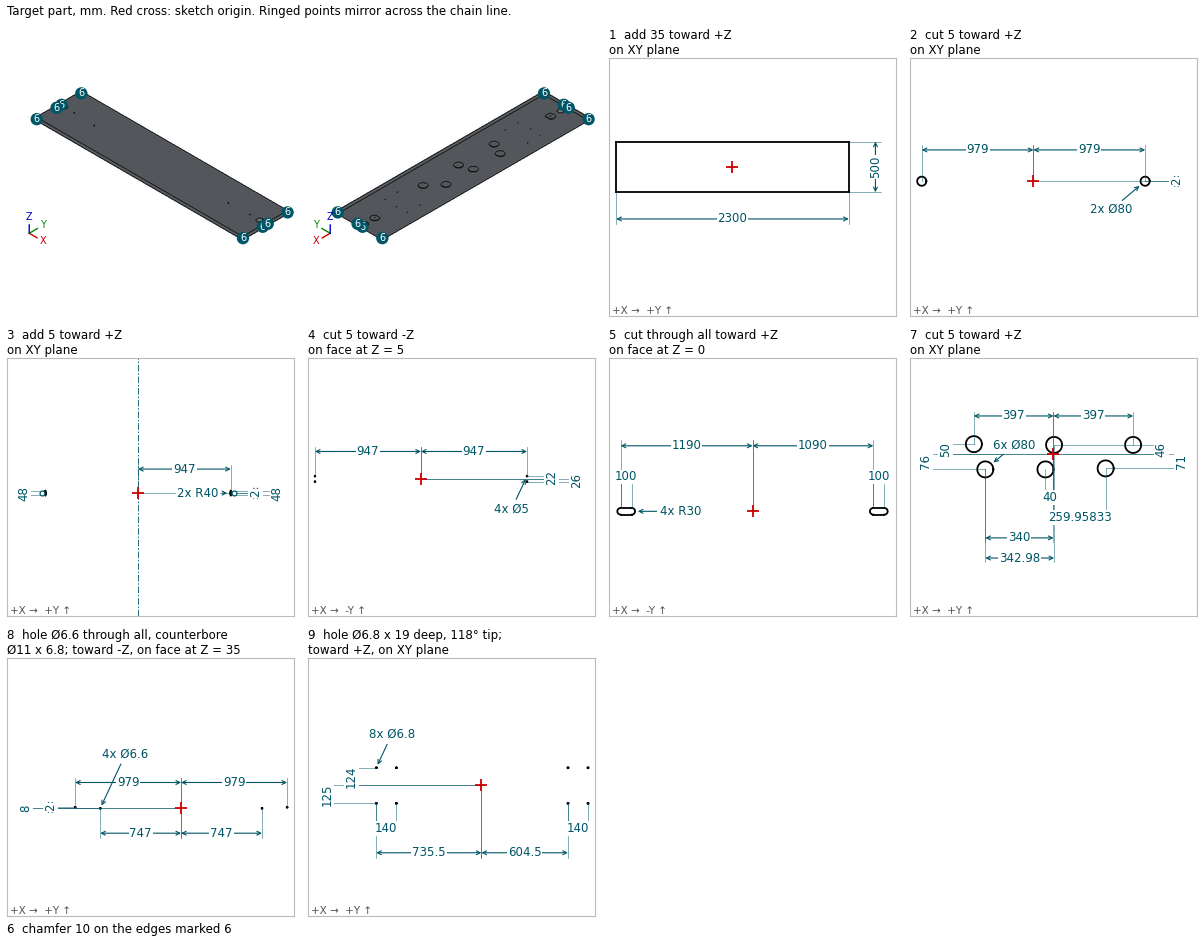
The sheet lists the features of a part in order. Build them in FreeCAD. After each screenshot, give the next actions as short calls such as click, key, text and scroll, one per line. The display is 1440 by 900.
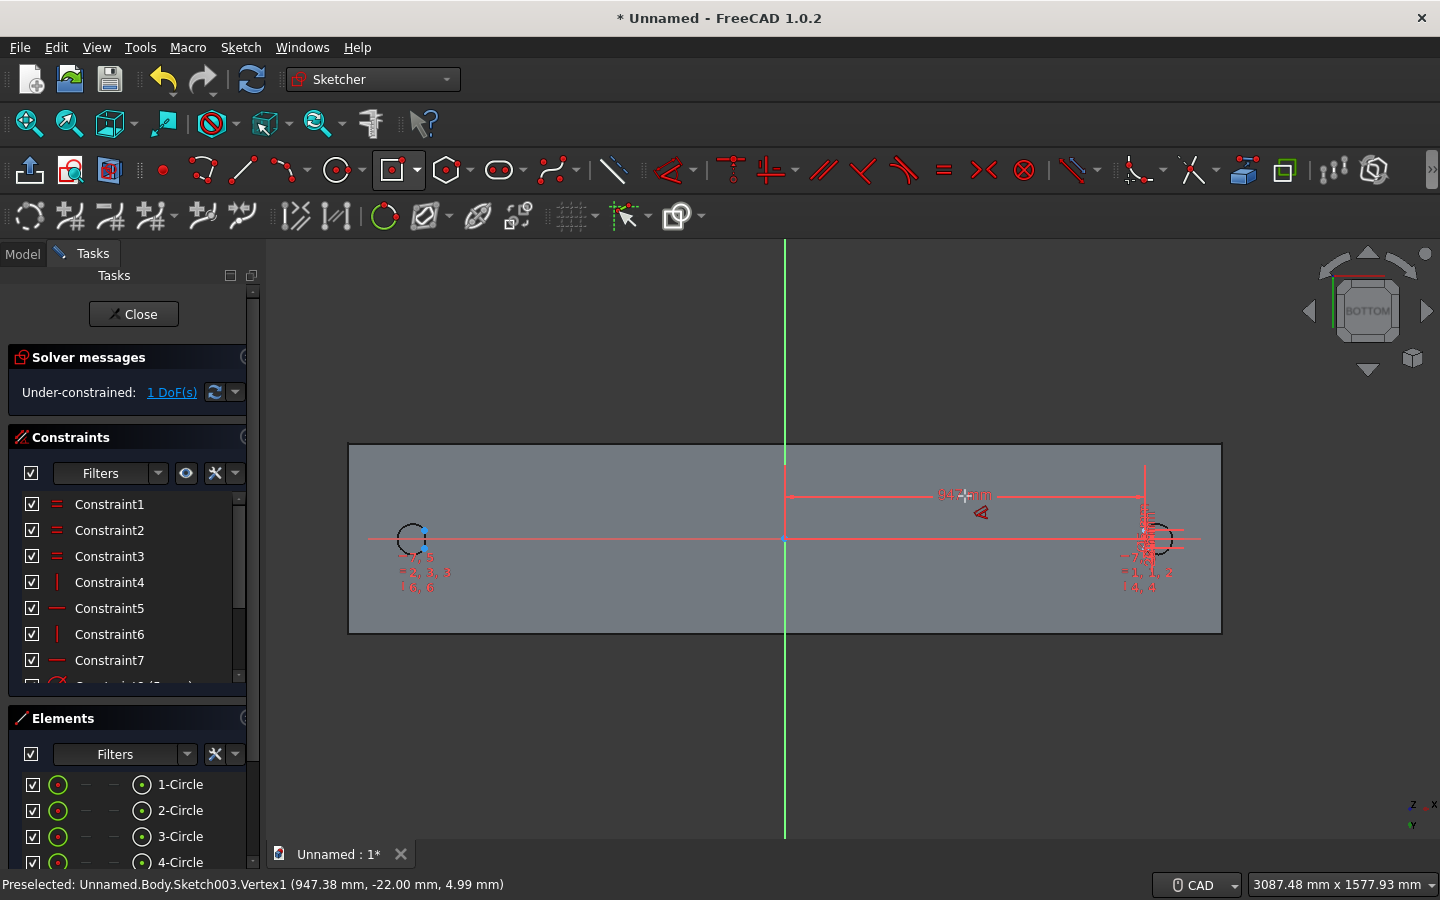
click(425, 530)
click(605, 496)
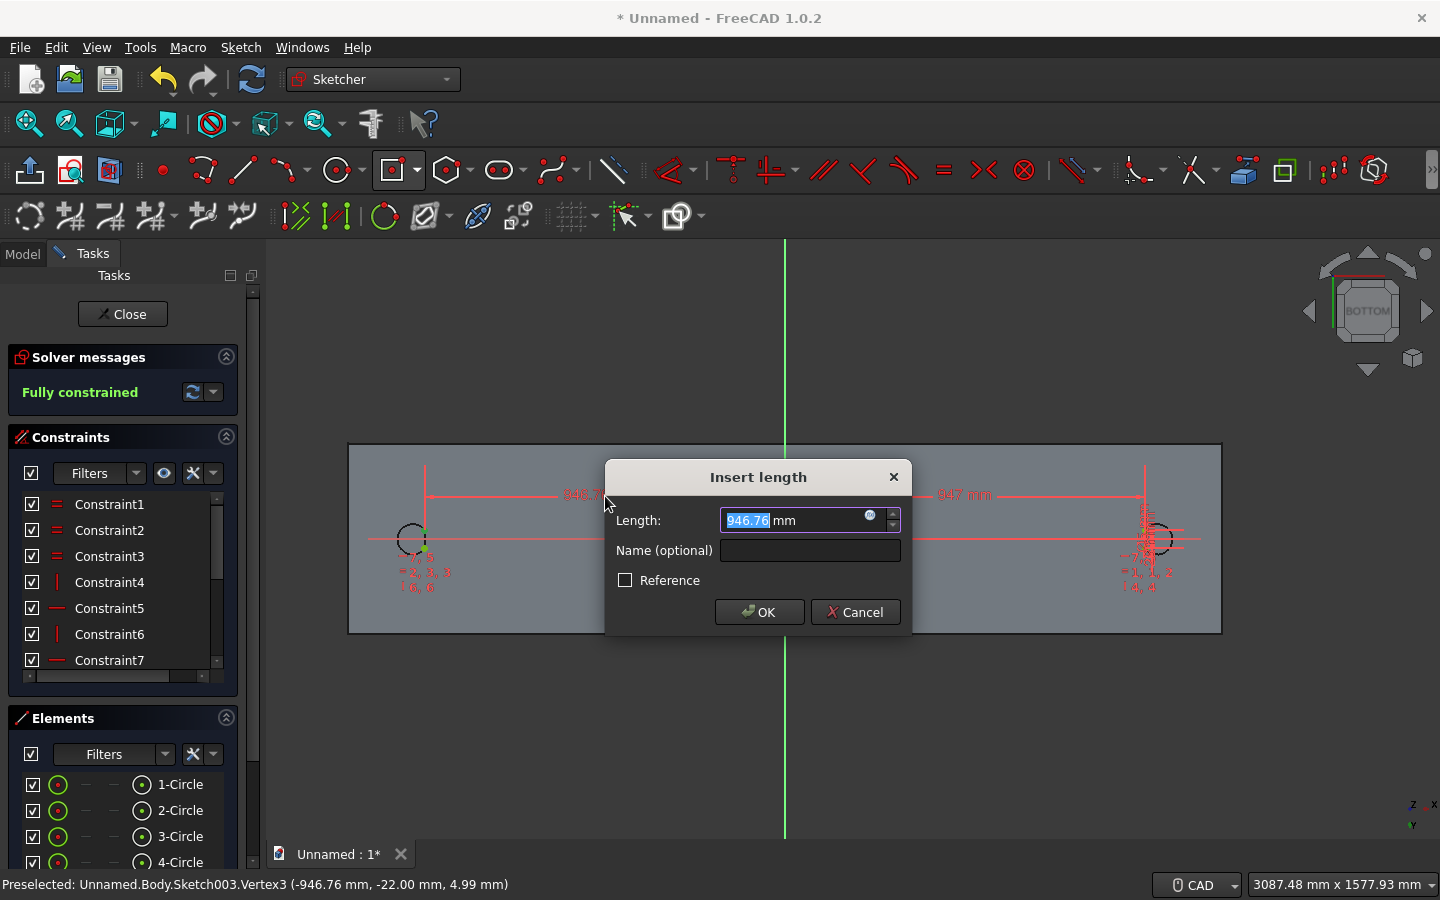
text(947)
key(Return)
key(Escape)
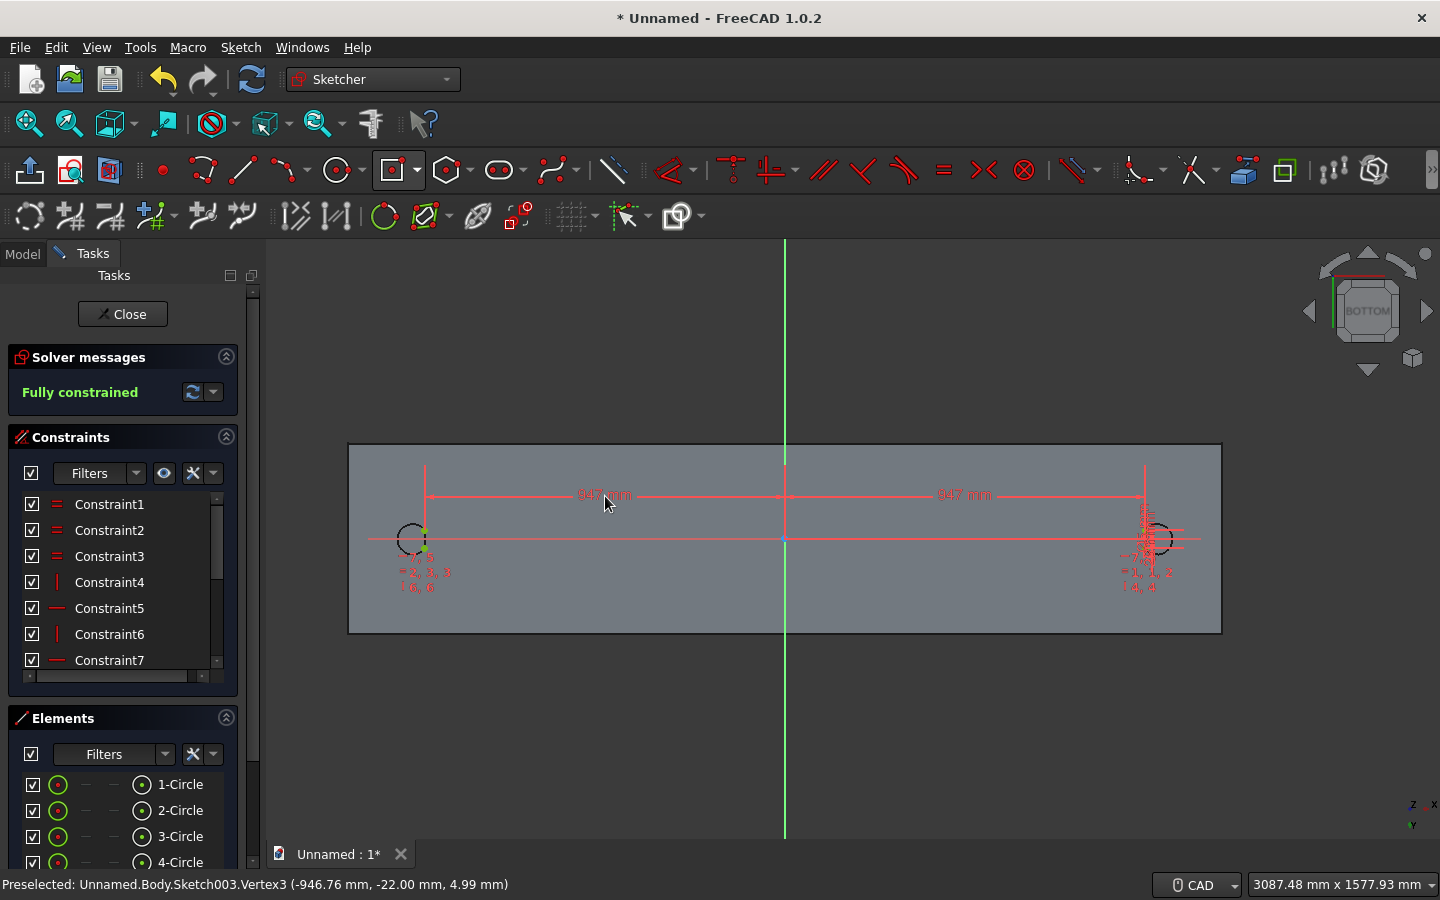
click(123, 314)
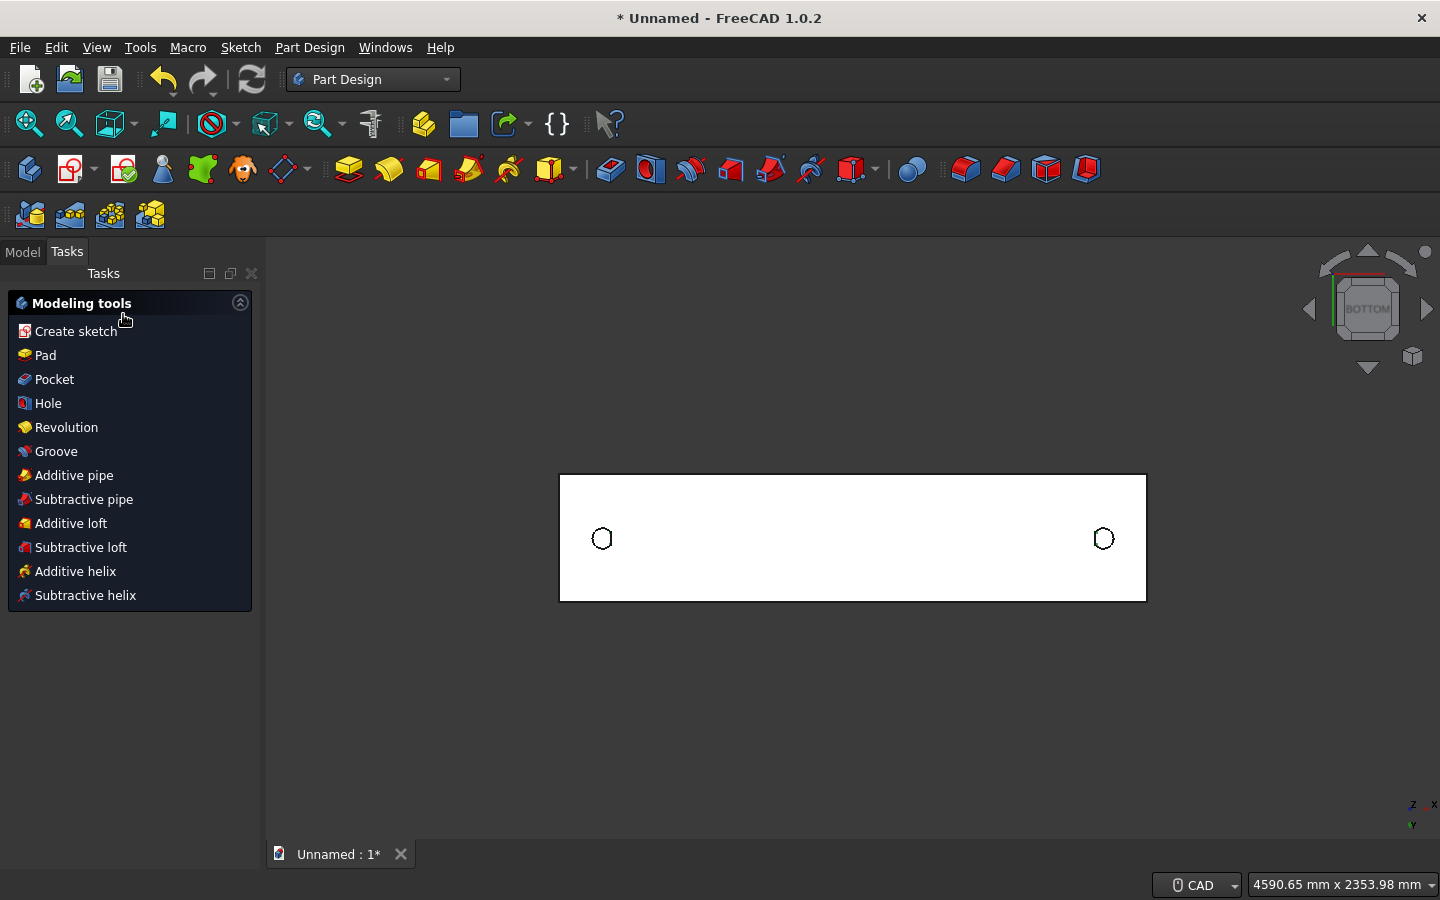
click(612, 170)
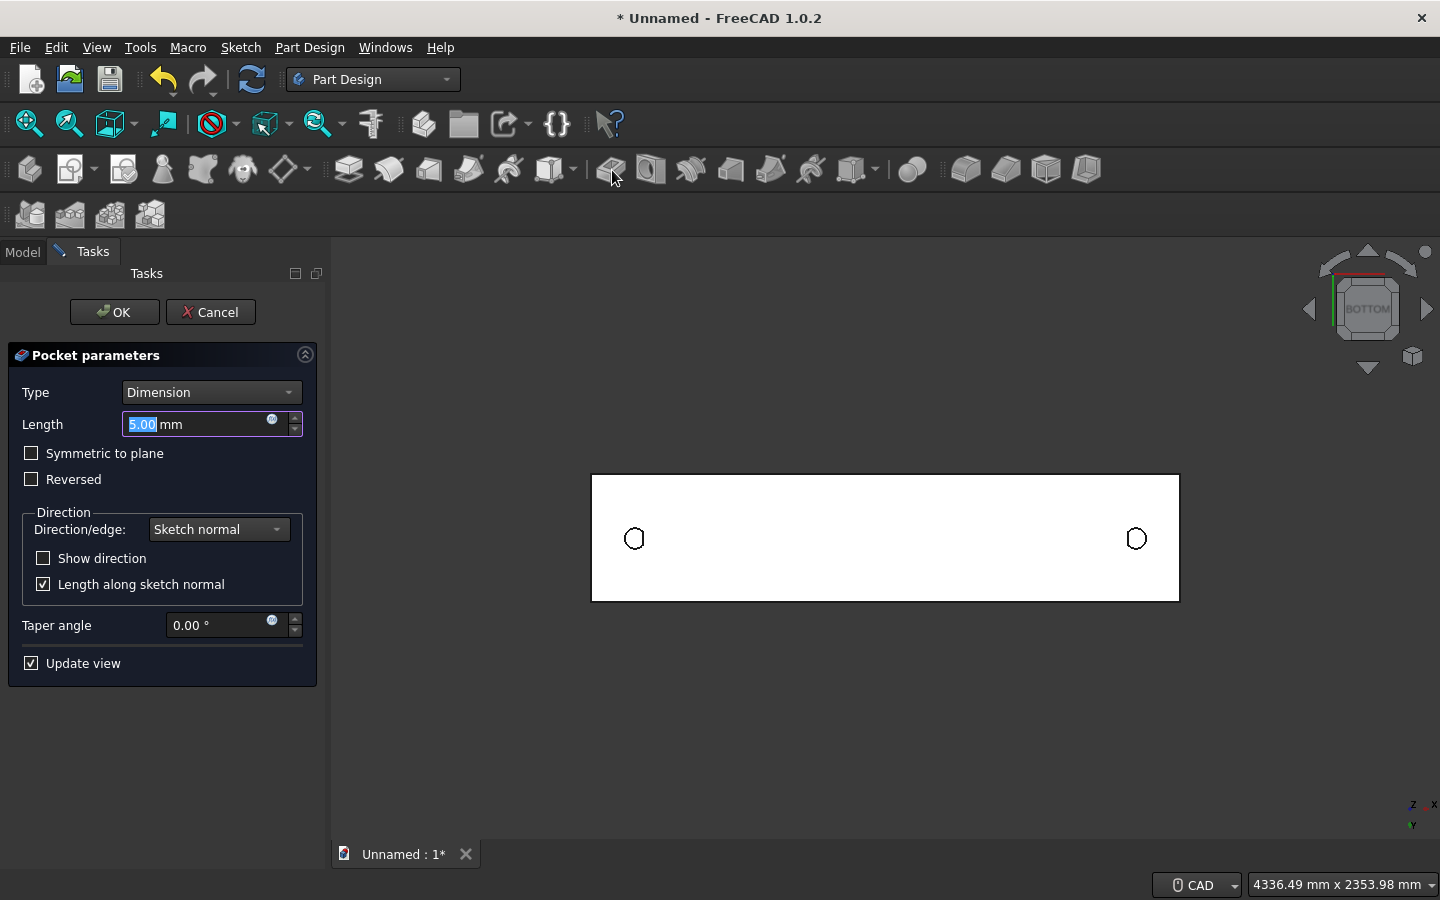
text(5)
key(Tab)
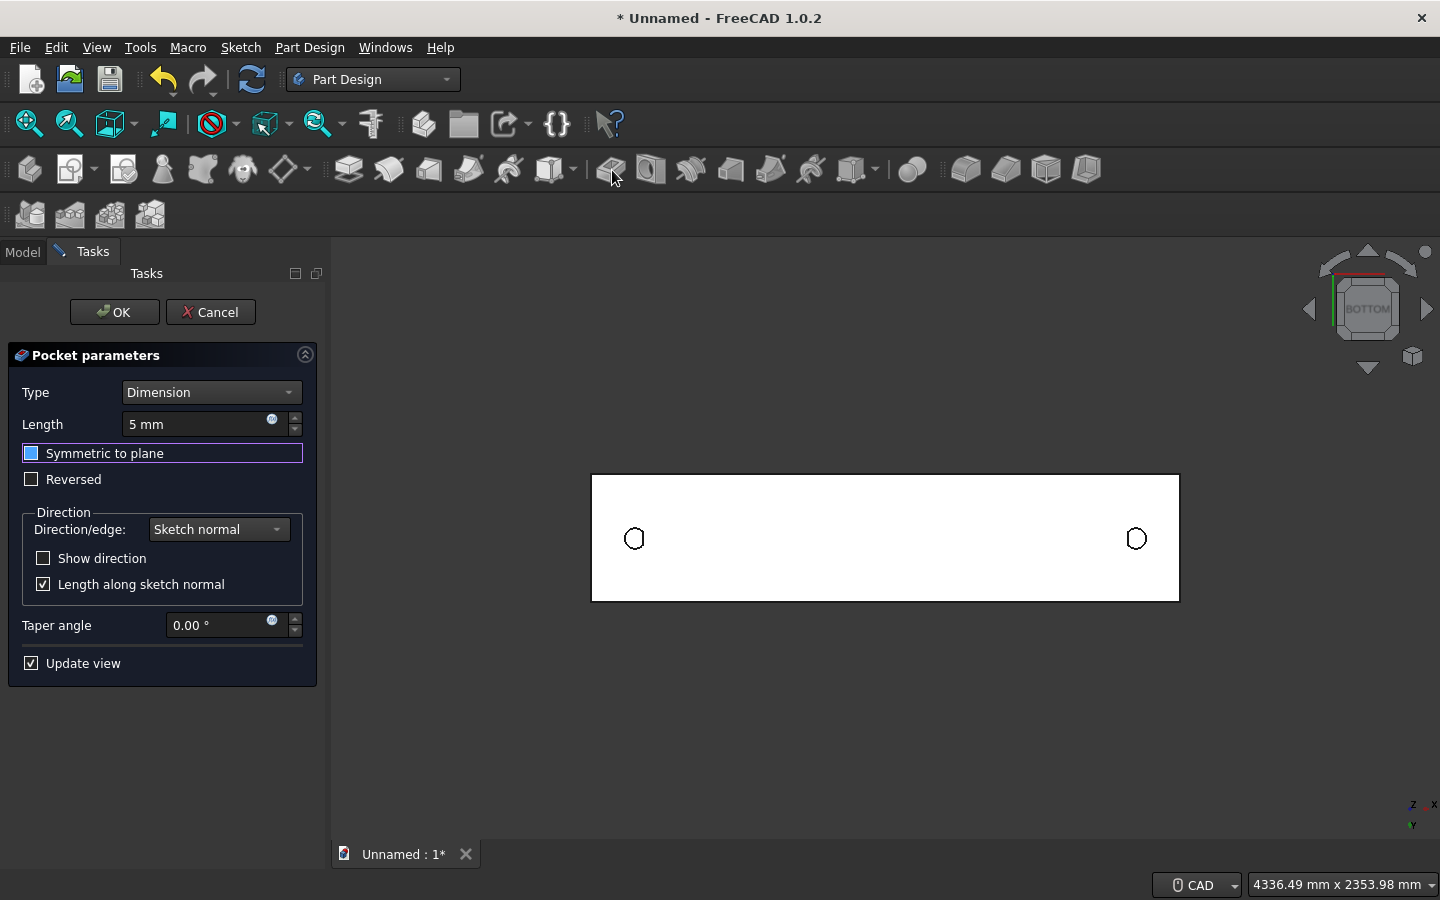
click(30, 479)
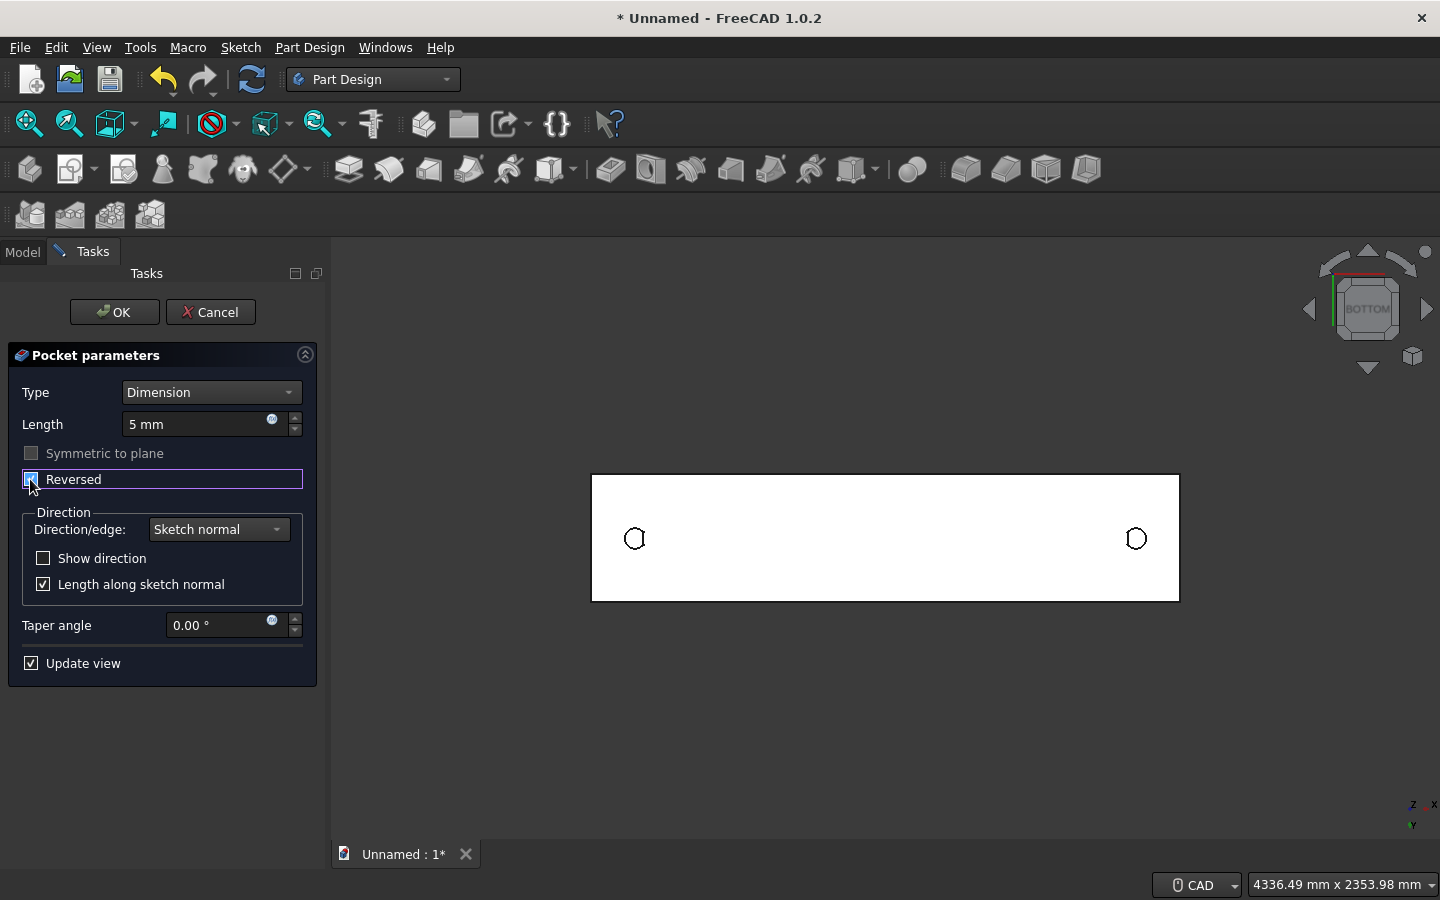
click(115, 312)